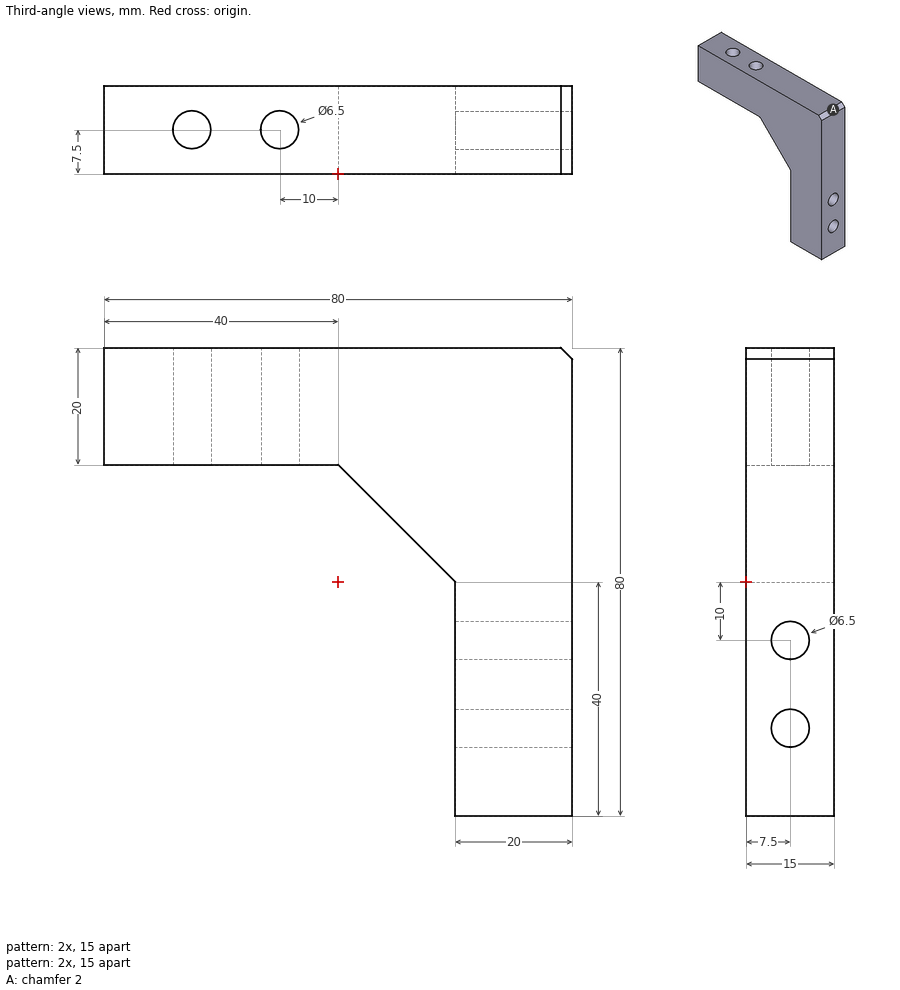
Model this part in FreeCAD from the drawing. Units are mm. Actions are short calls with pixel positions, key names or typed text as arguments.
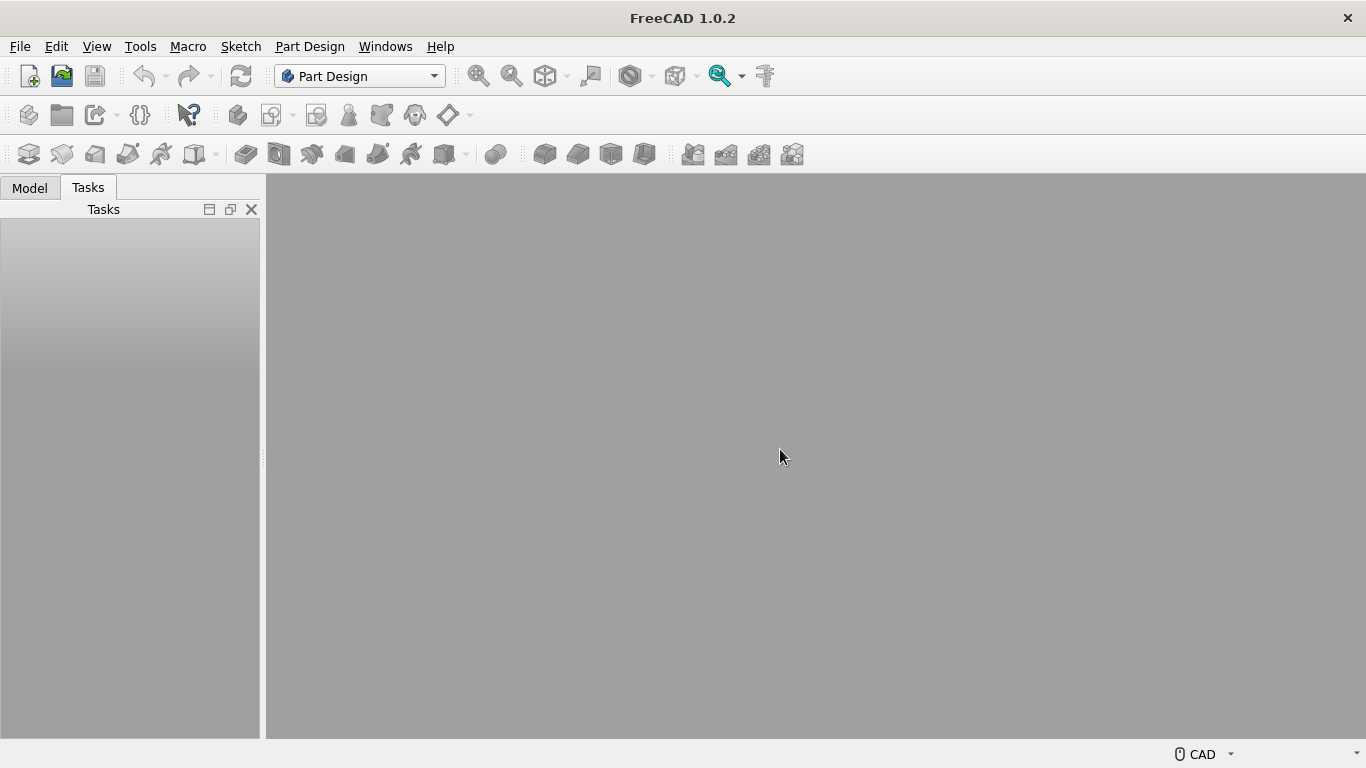
key(ctrl+n)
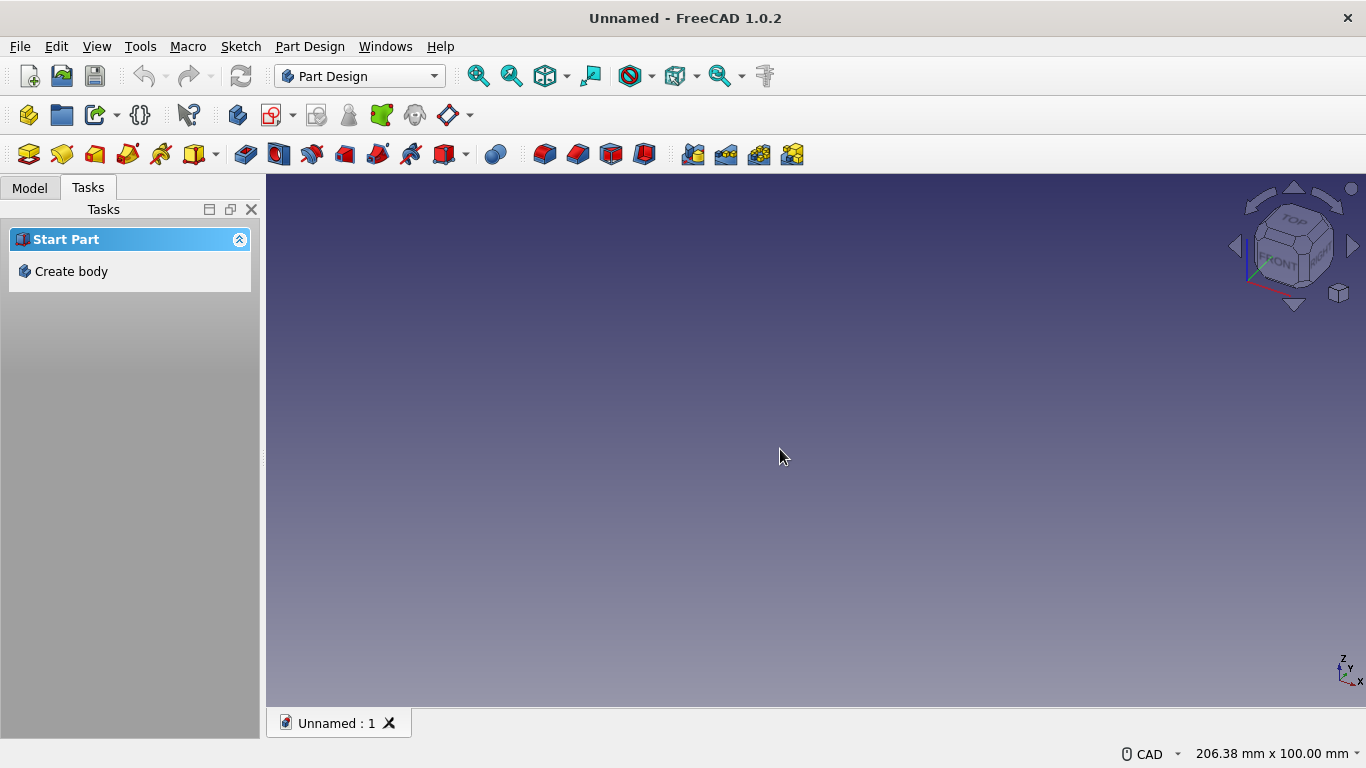
click(270, 116)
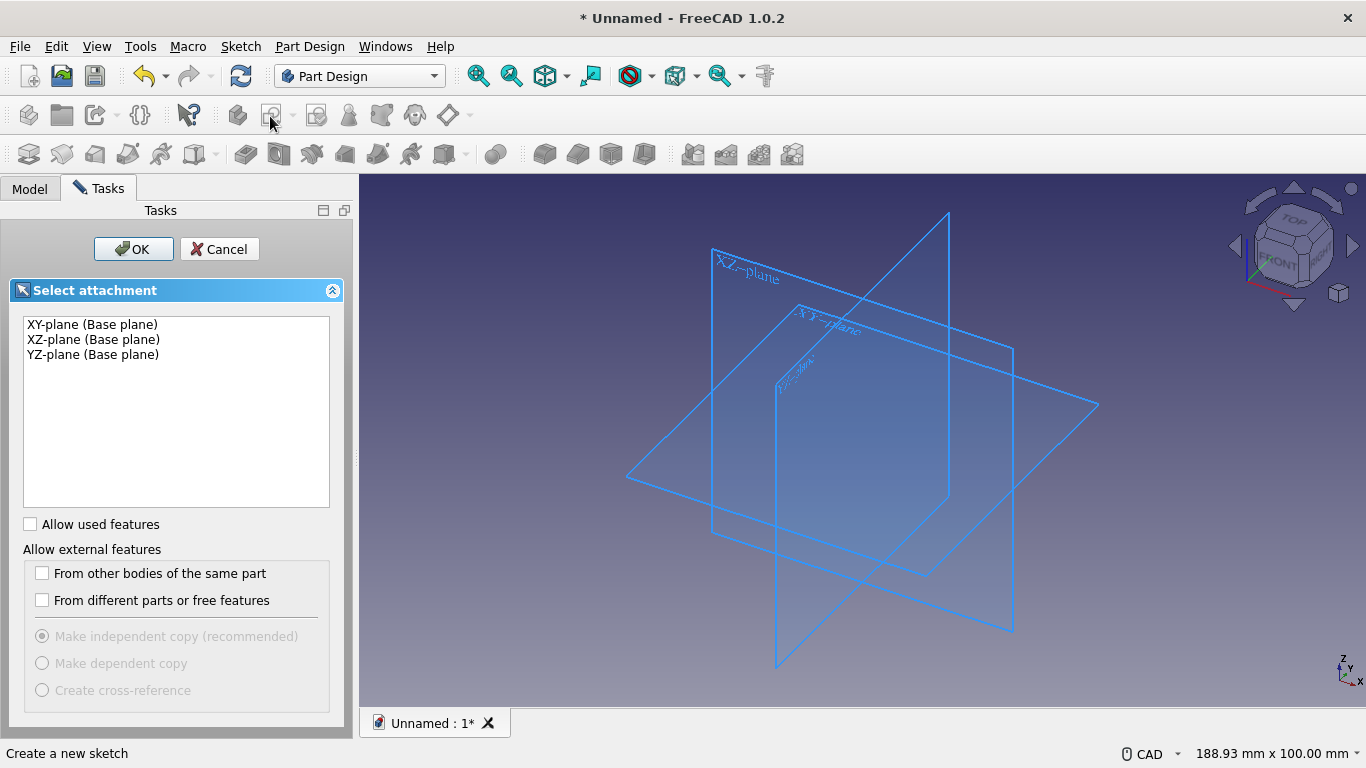
click(84, 340)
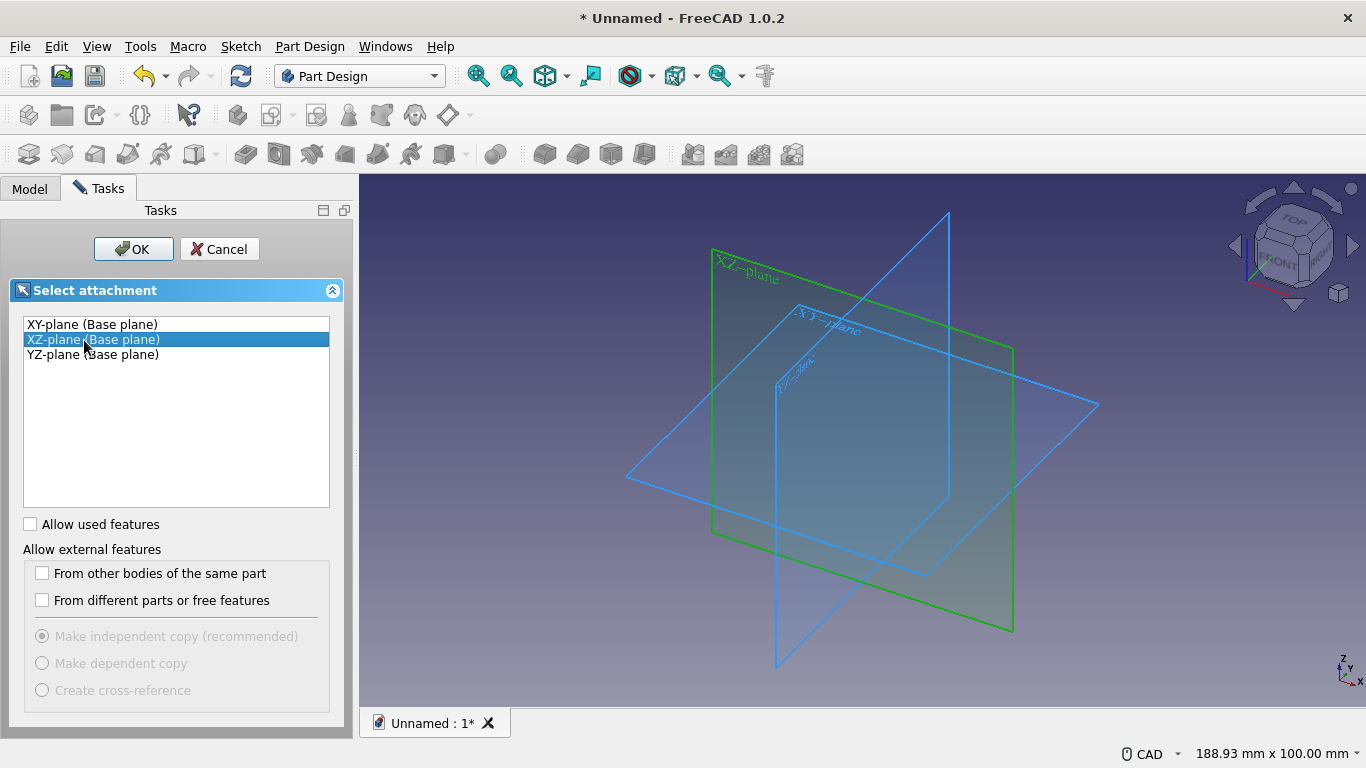
click(134, 249)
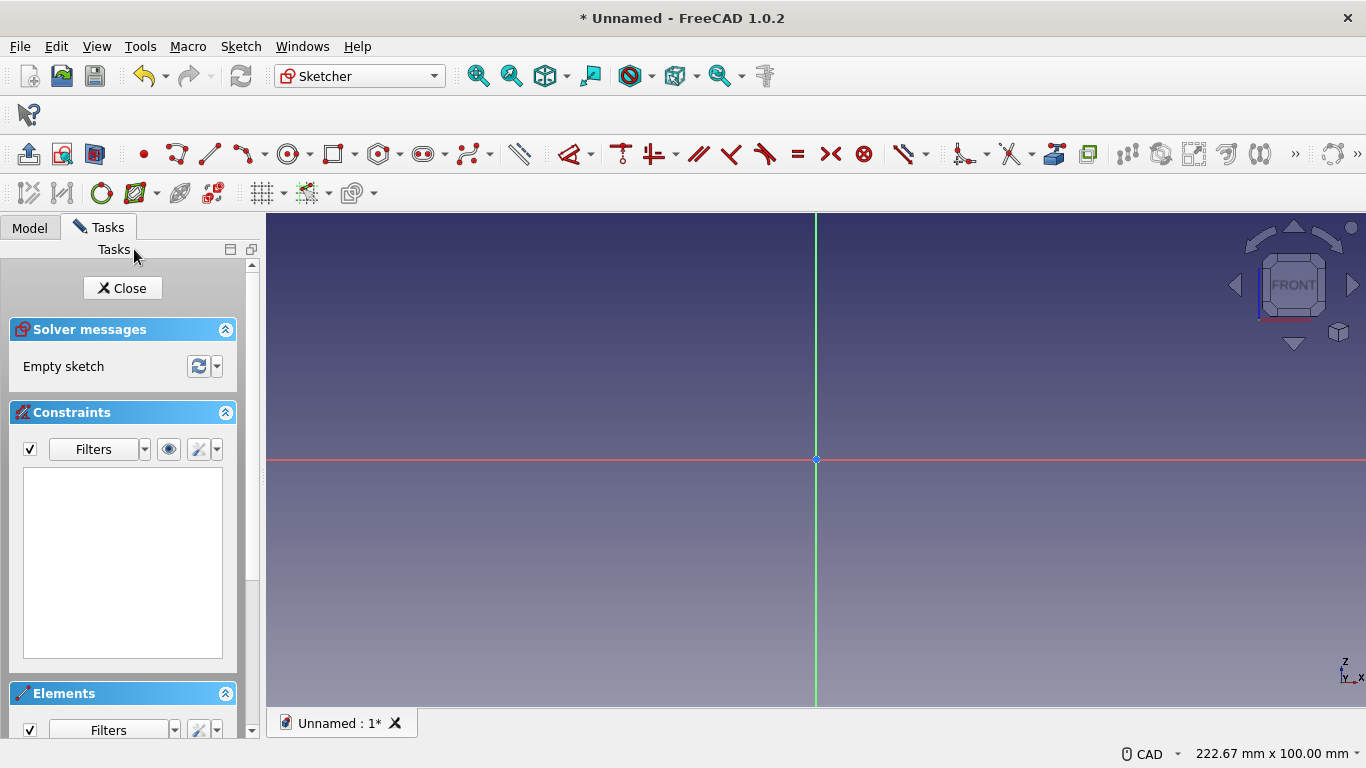
scroll(438, 460, down, 1)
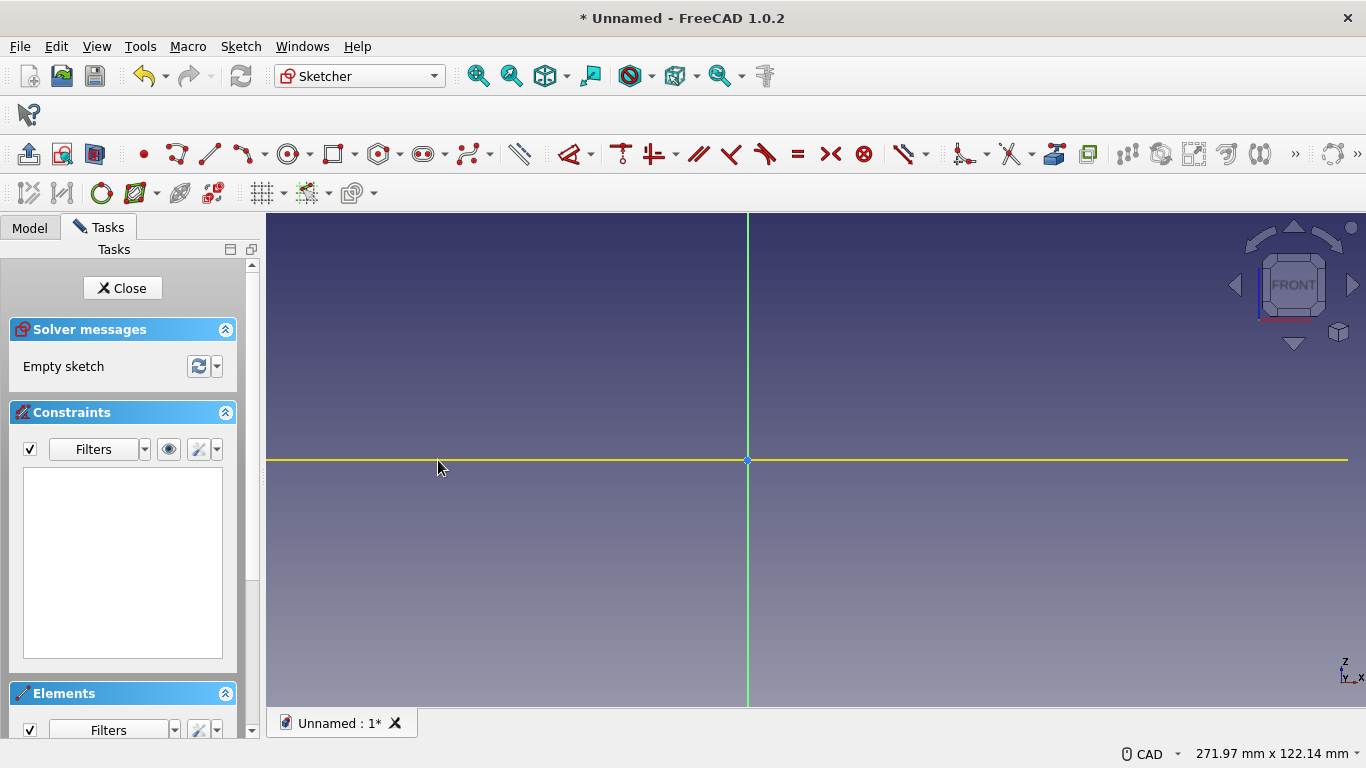
click(177, 154)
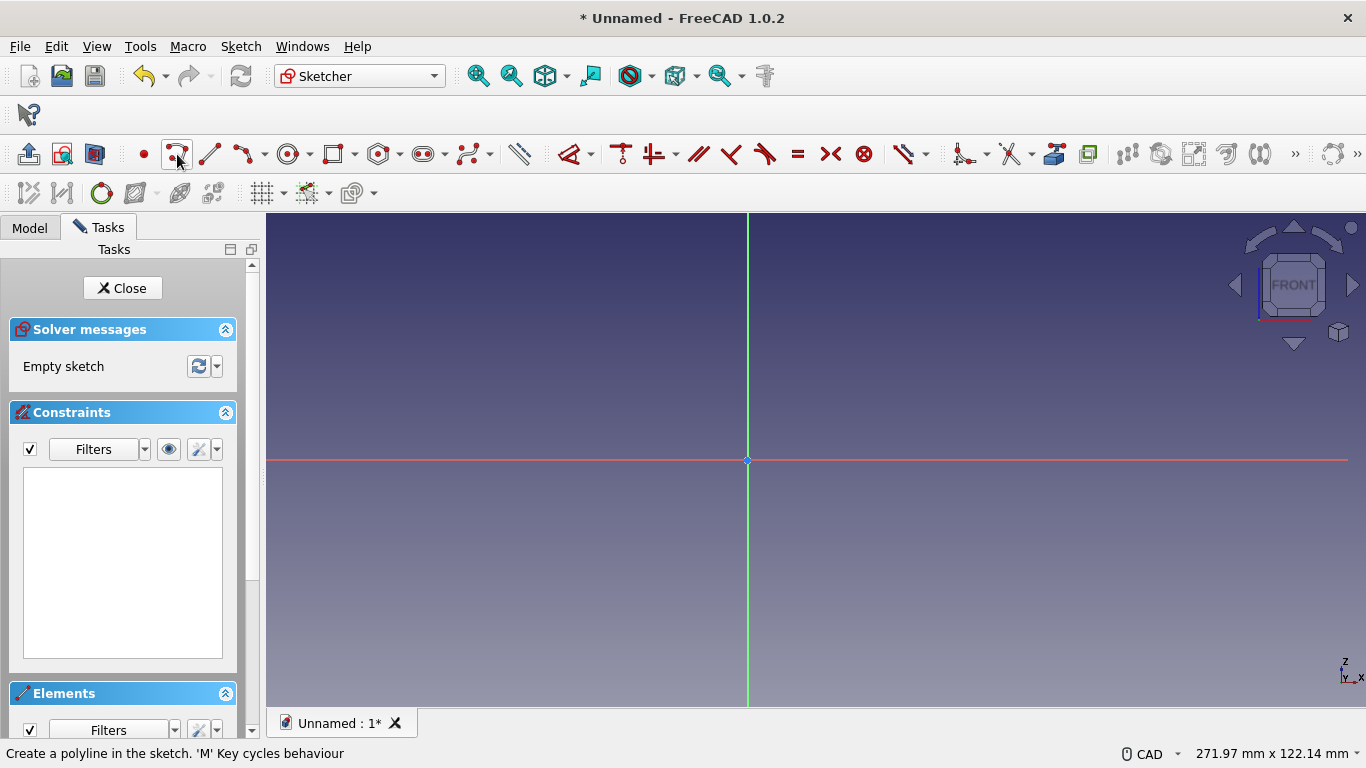
click(828, 460)
click(748, 379)
click(586, 379)
click(586, 298)
click(909, 298)
click(909, 622)
click(828, 622)
click(828, 460)
key(Escape)
key(Escape)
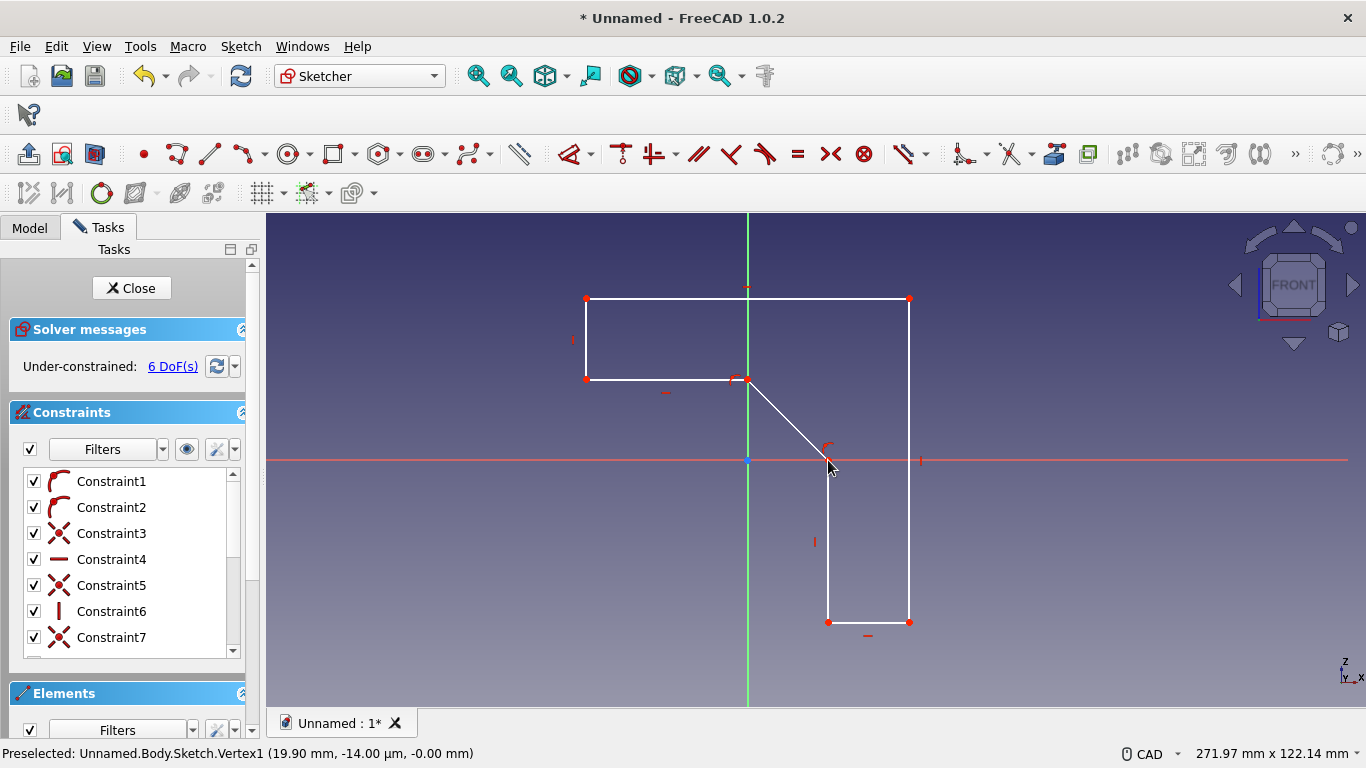
key(d)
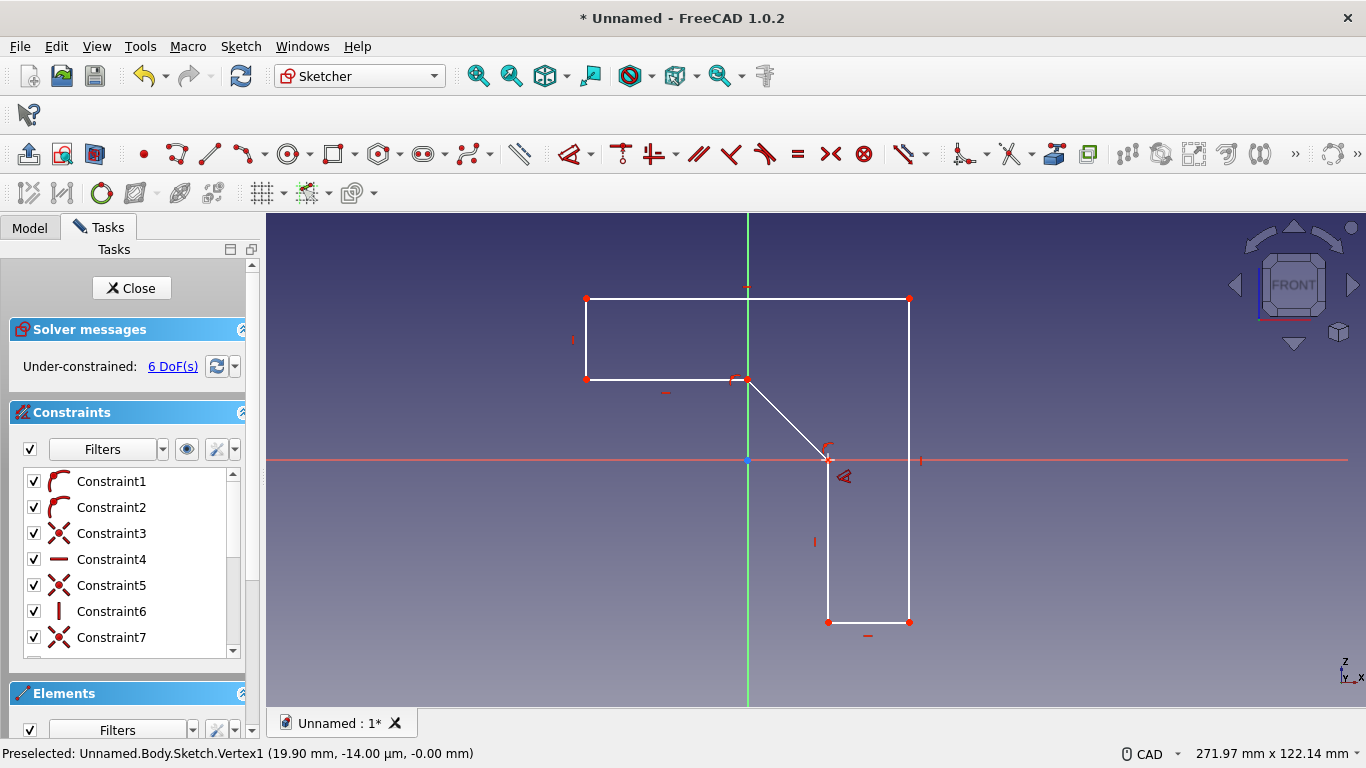
click(699, 380)
click(667, 346)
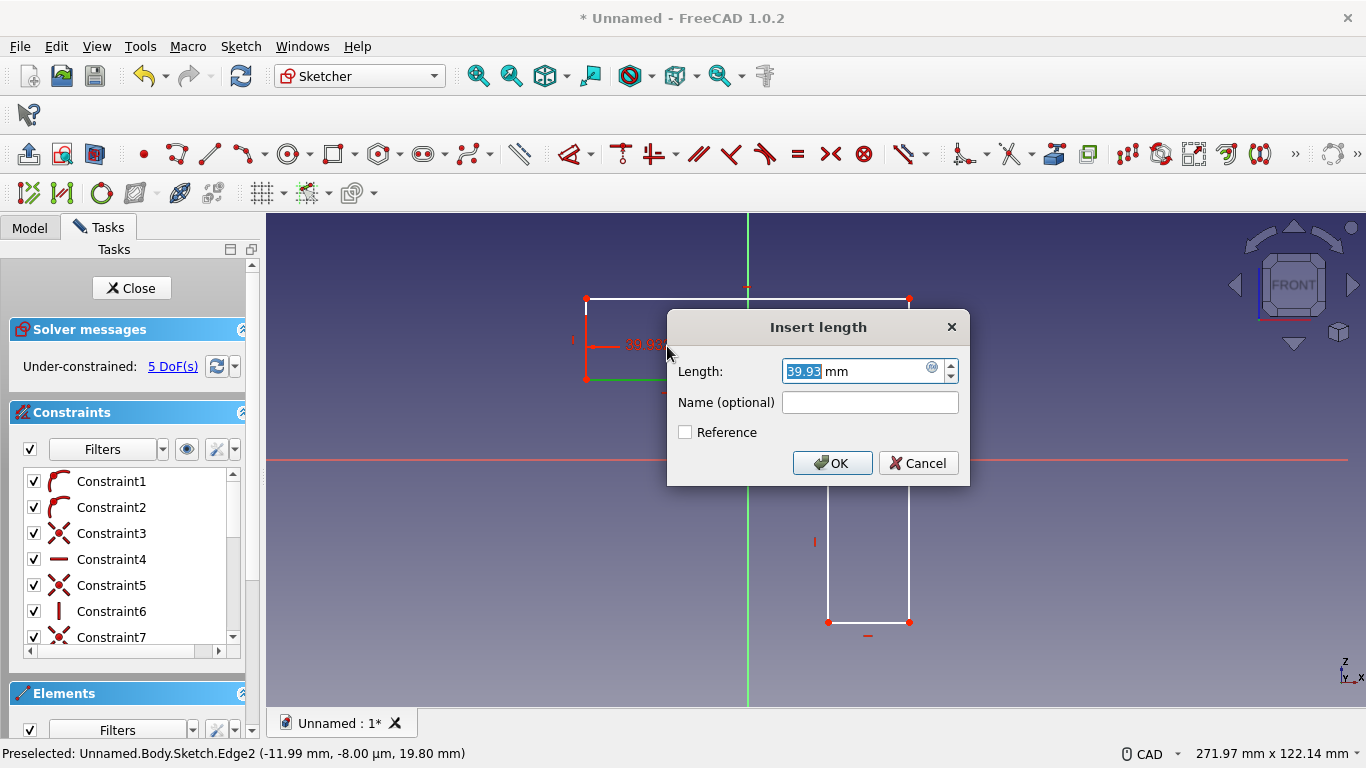
text(40)
key(Return)